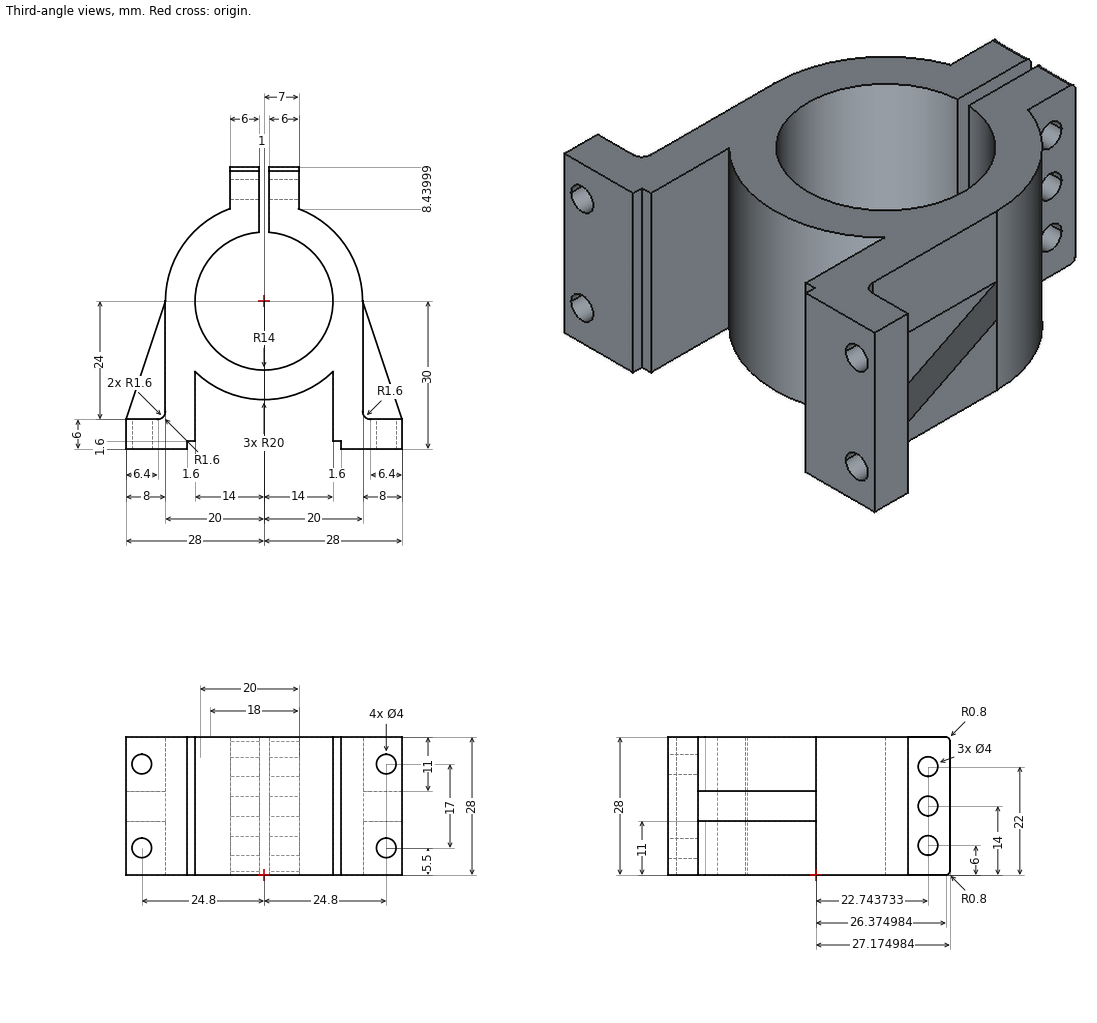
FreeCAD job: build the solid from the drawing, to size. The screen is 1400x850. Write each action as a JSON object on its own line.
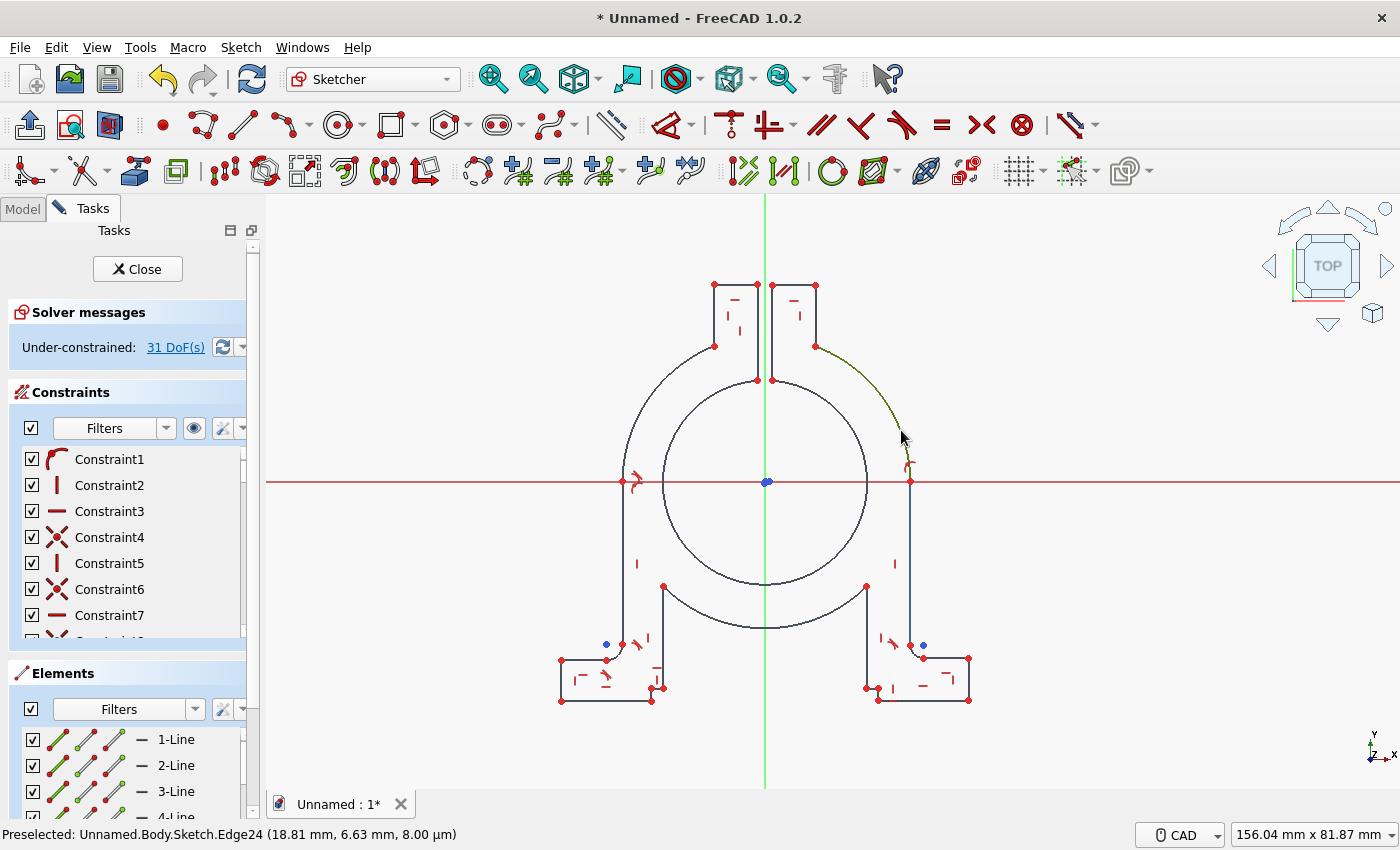
{"action": "left_click", "coordinate": [902, 126]}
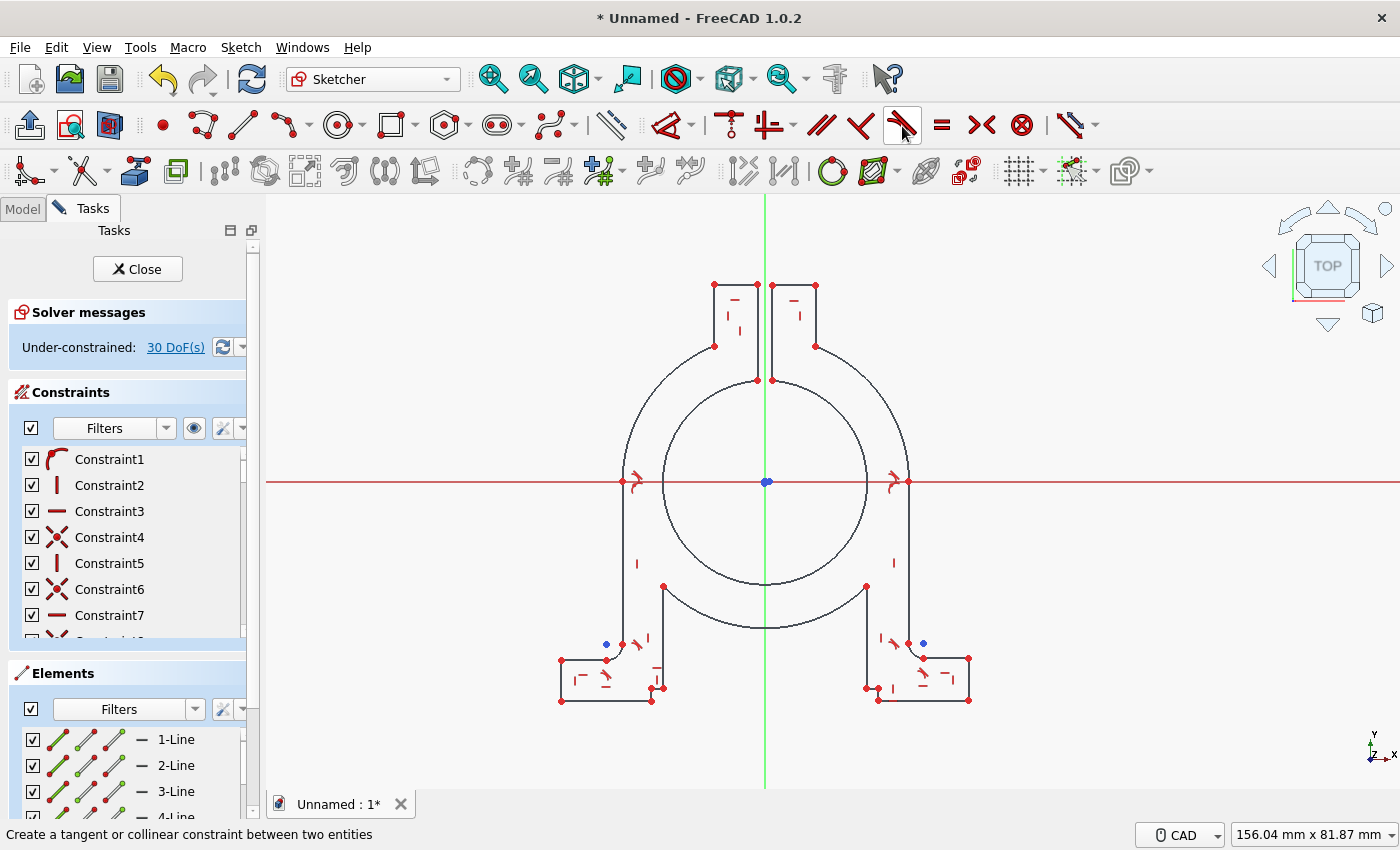
{"action": "left_click", "coordinate": [720, 621]}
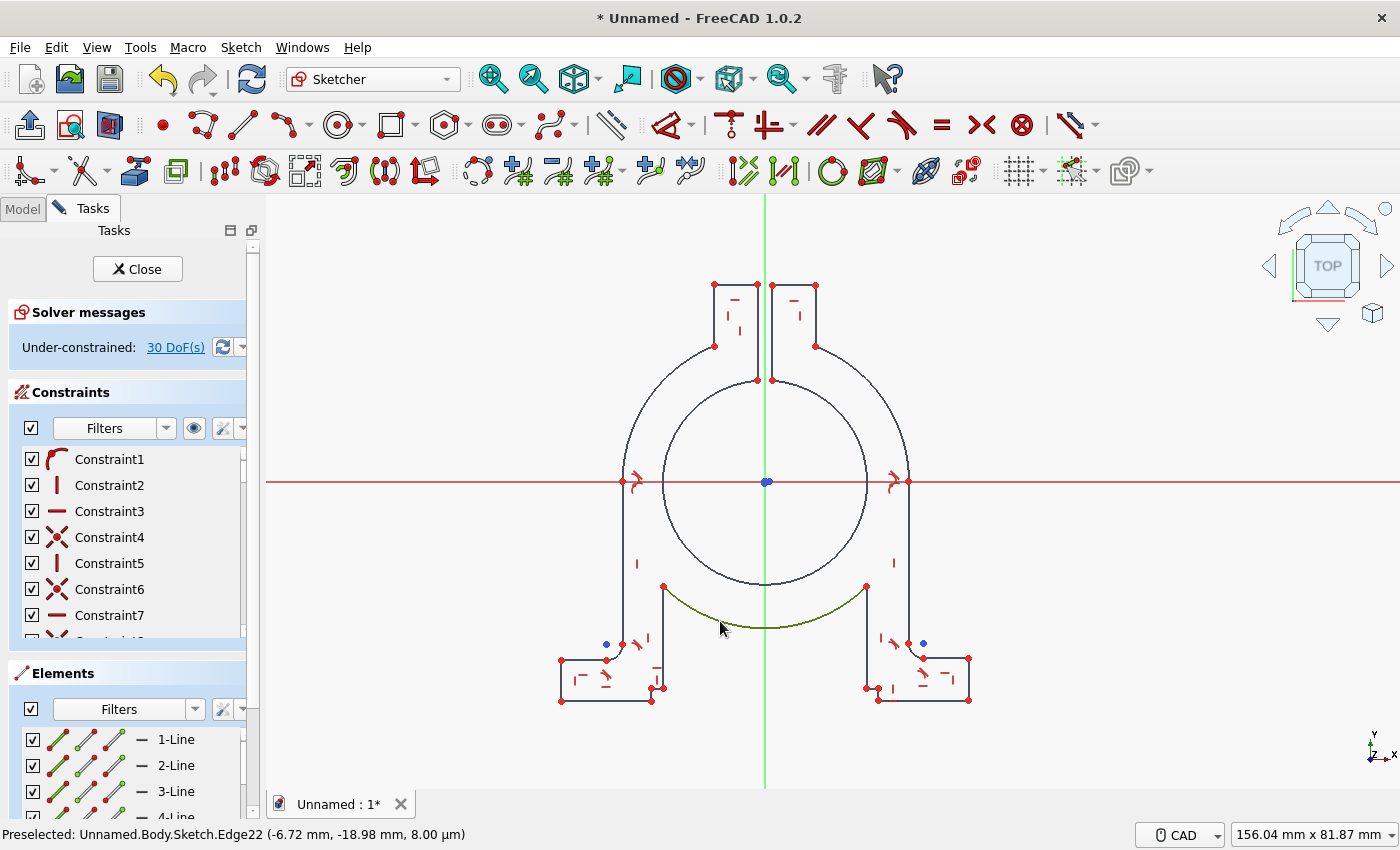
{"action": "left_click", "coordinate": [900, 431]}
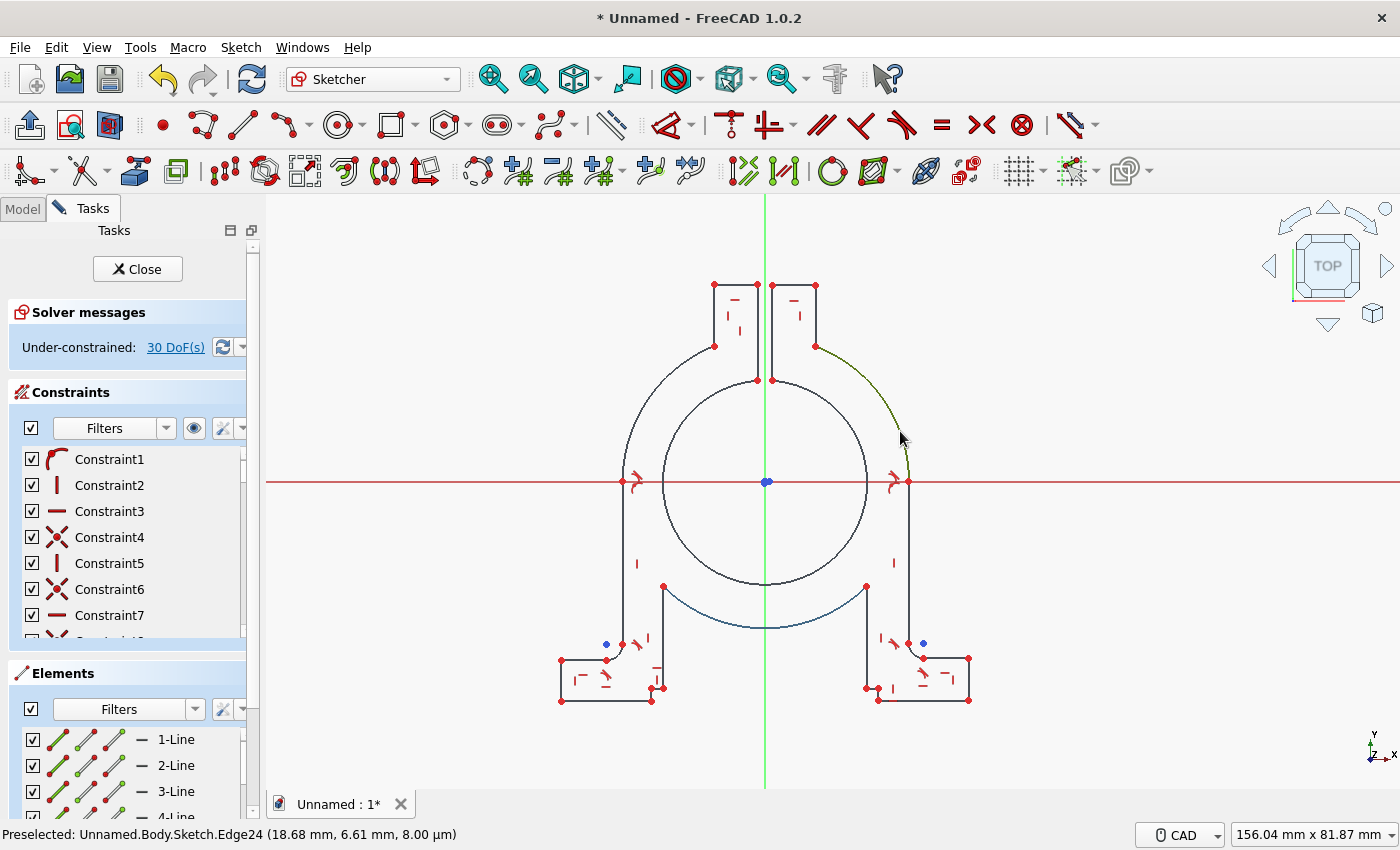
{"action": "left_click", "coordinate": [730, 126]}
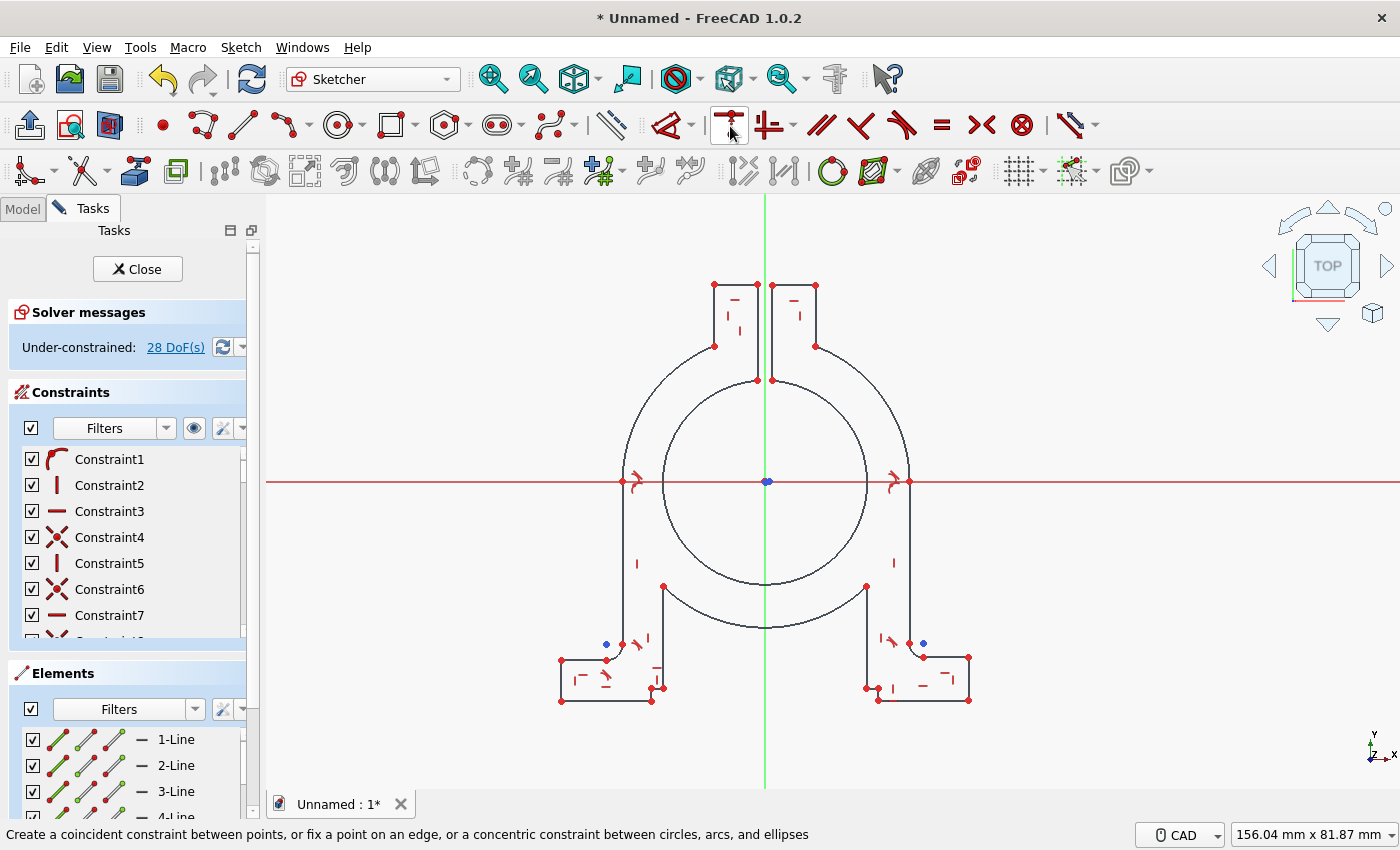
{"action": "left_click", "coordinate": [721, 621]}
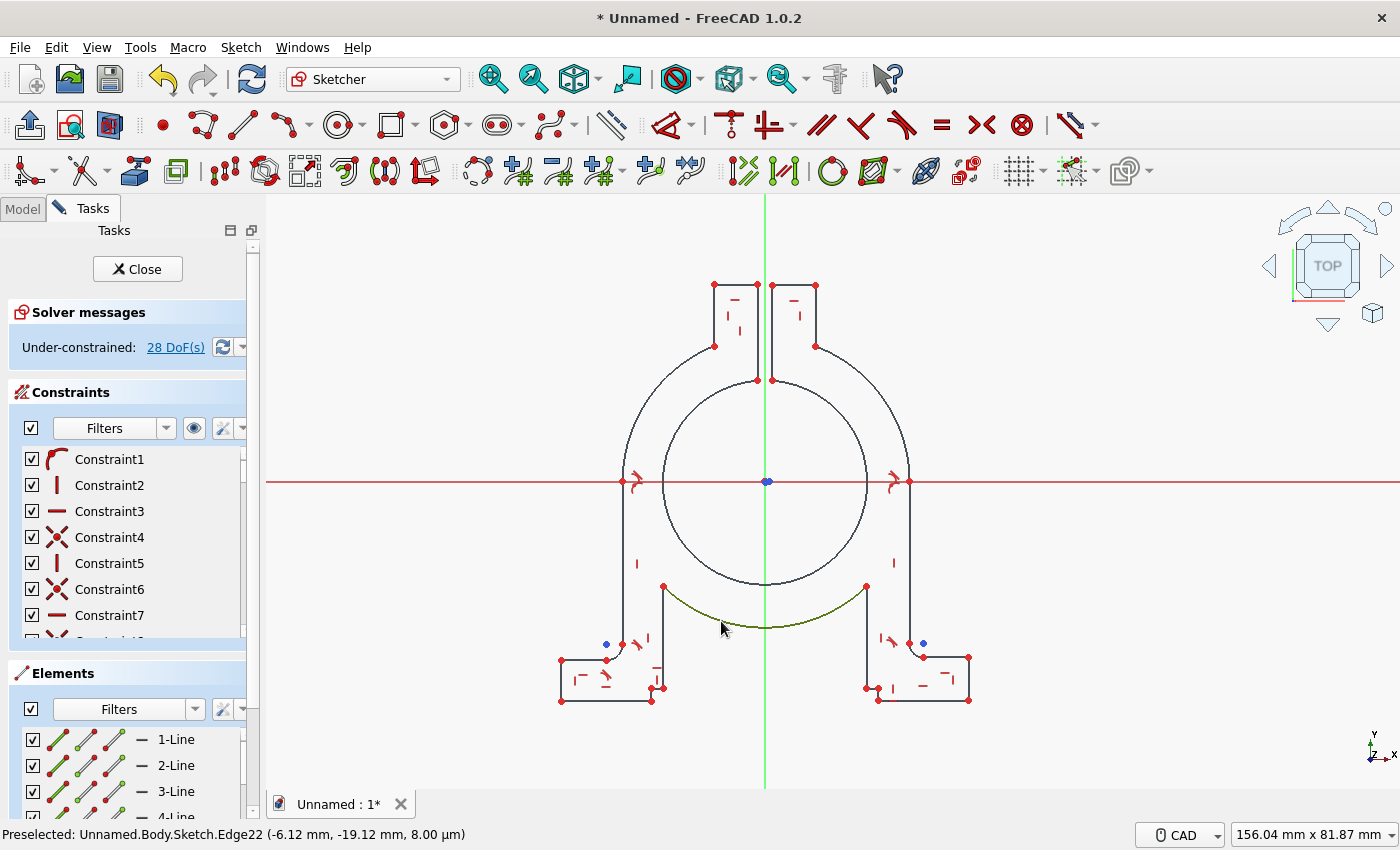
{"action": "left_click", "coordinate": [669, 517]}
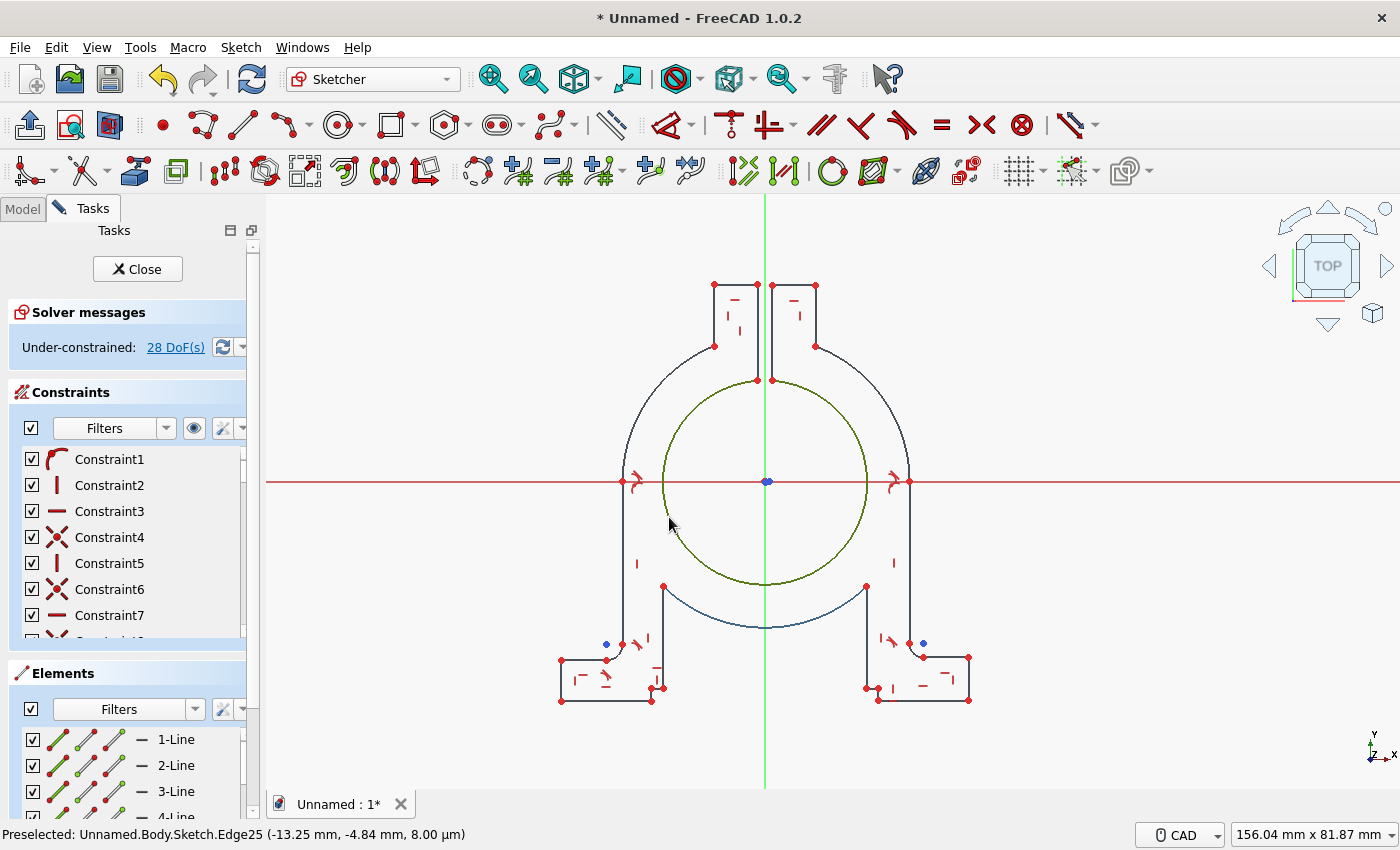
{"action": "left_click", "coordinate": [730, 126]}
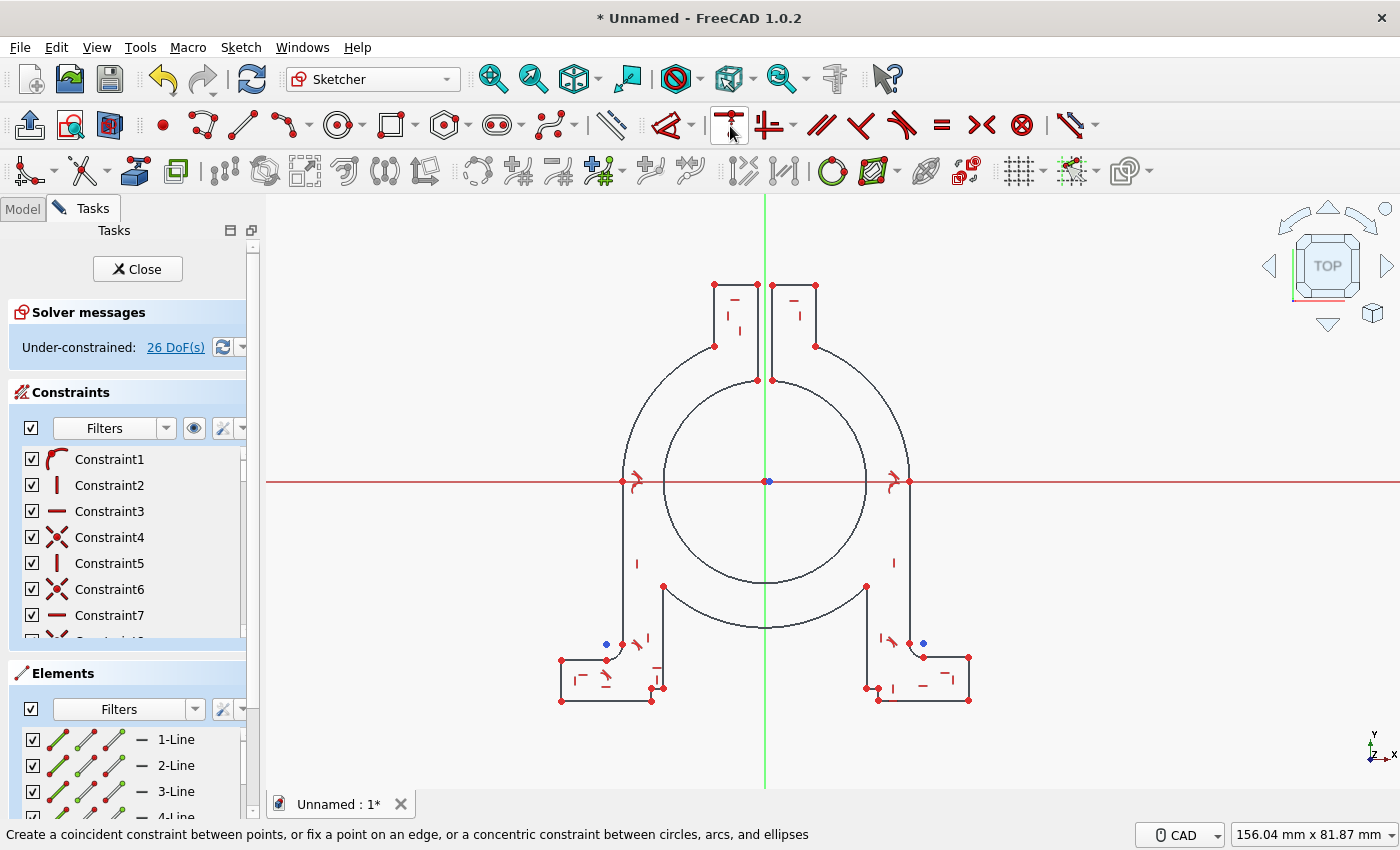
{"action": "left_click", "coordinate": [618, 655]}